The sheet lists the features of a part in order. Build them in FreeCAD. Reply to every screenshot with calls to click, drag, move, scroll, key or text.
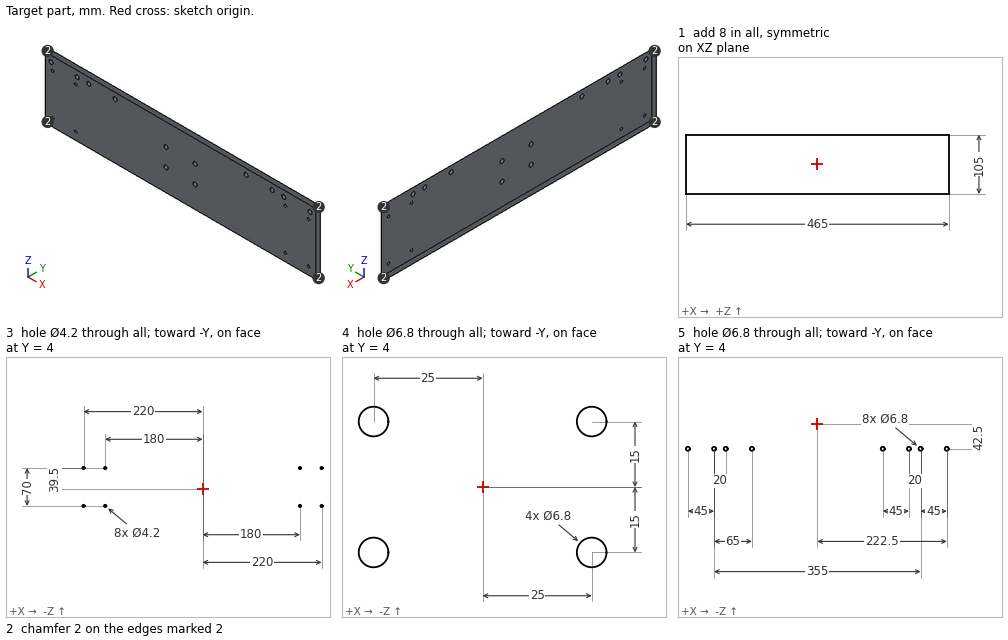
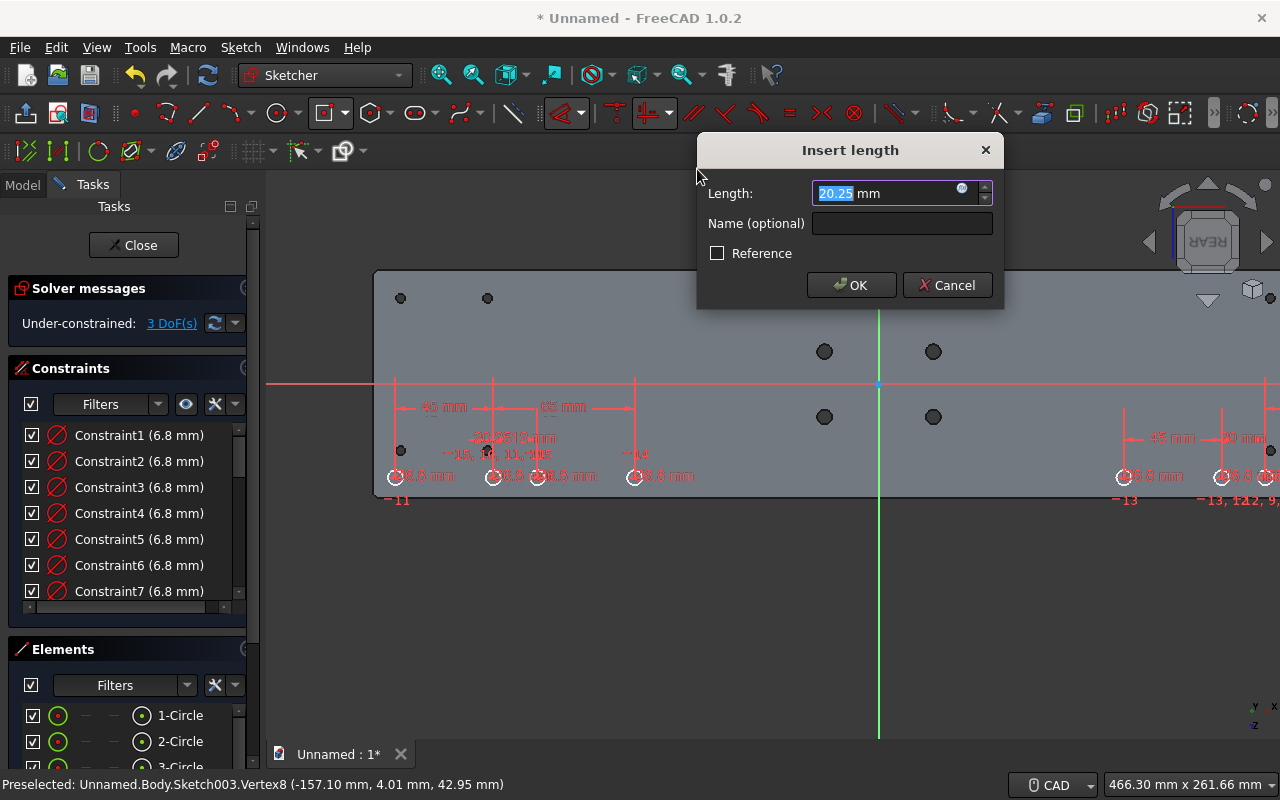
text(20)
key(Return)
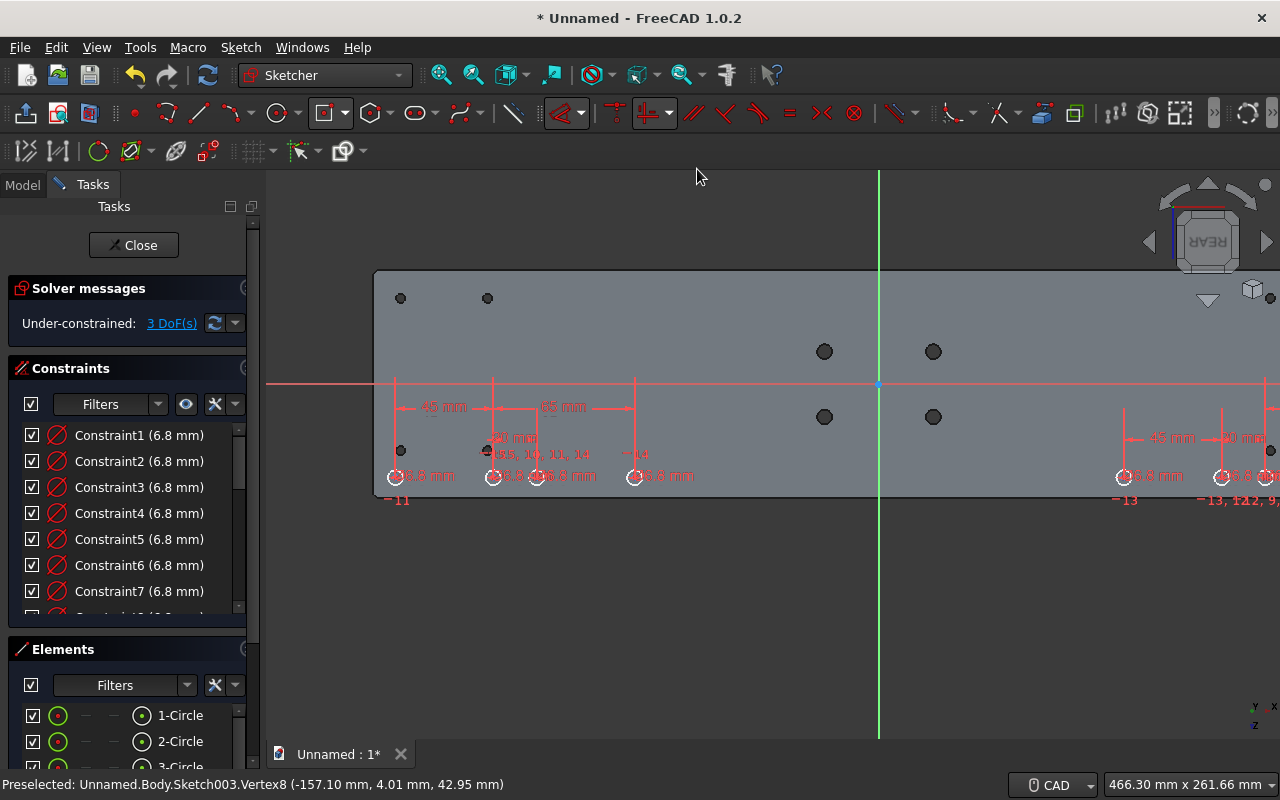
scroll(492, 479, down, 3)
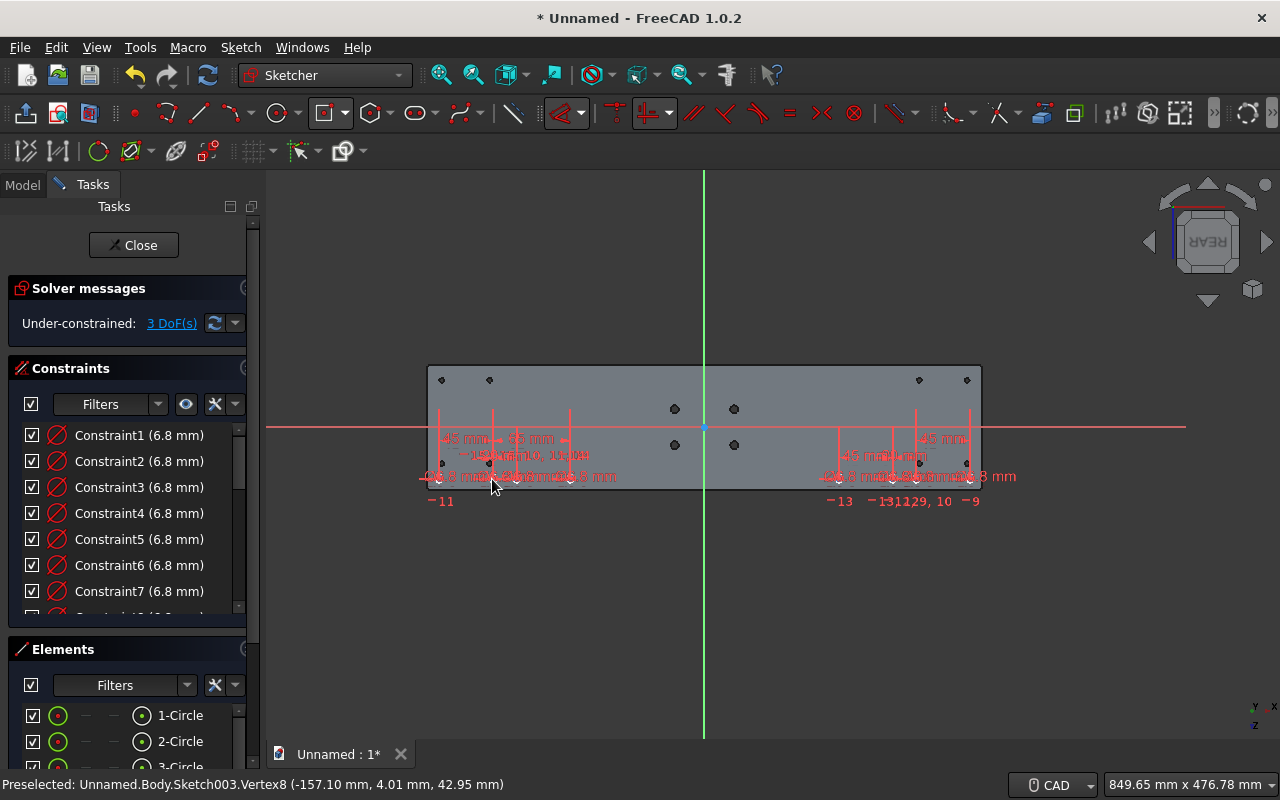
click(970, 479)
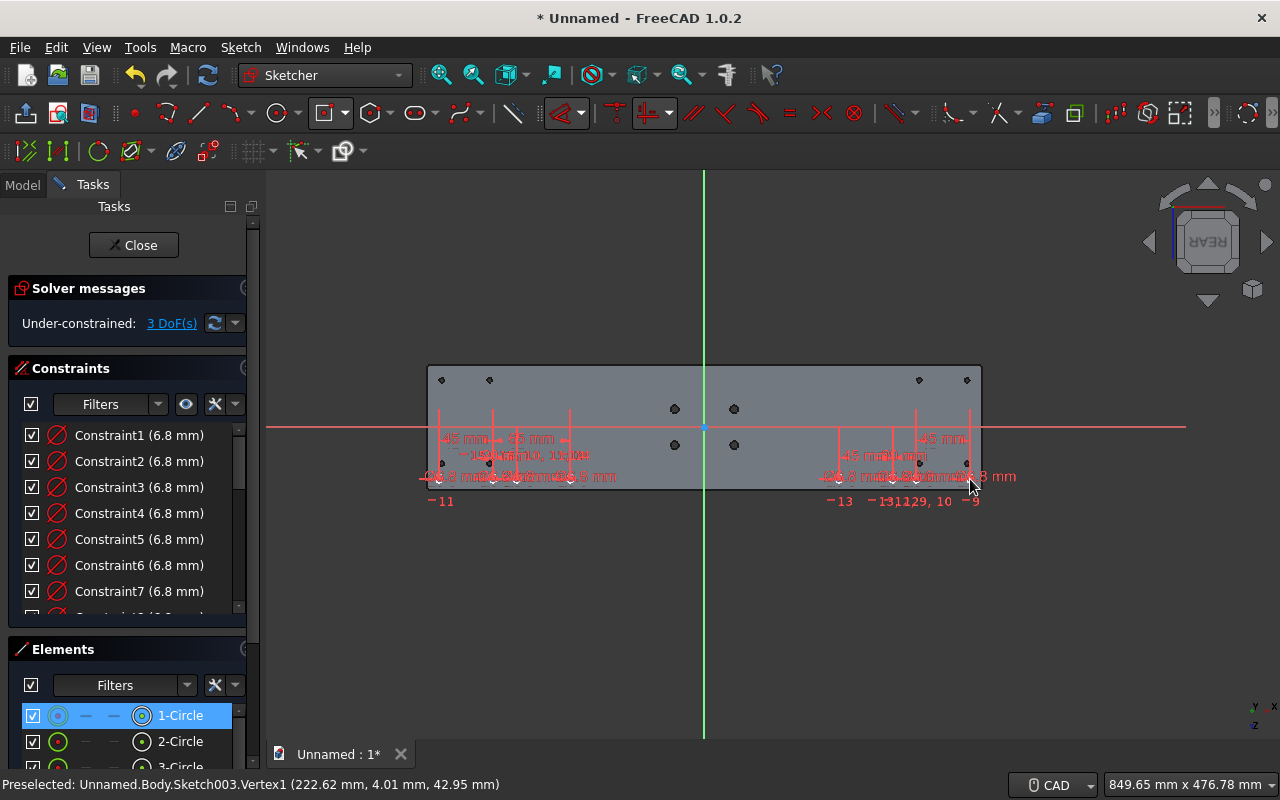
click(584, 114)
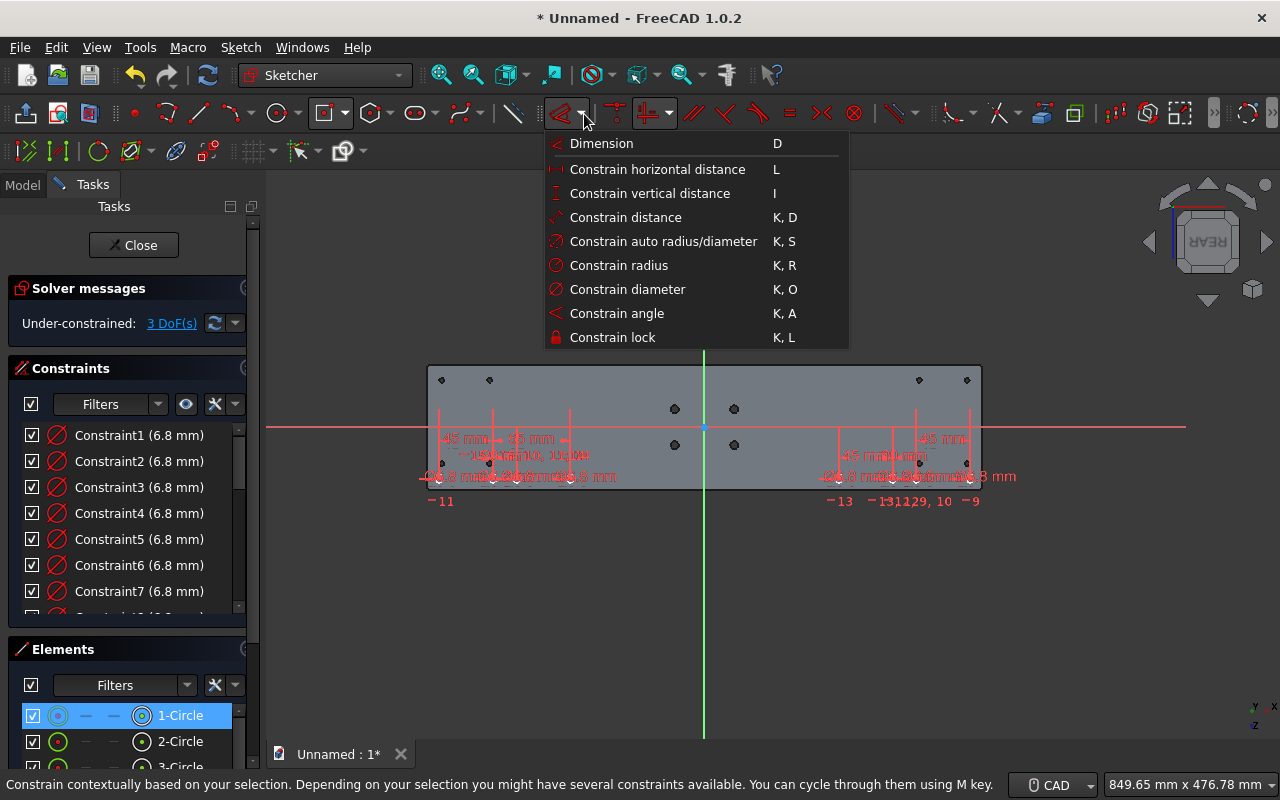
click(697, 193)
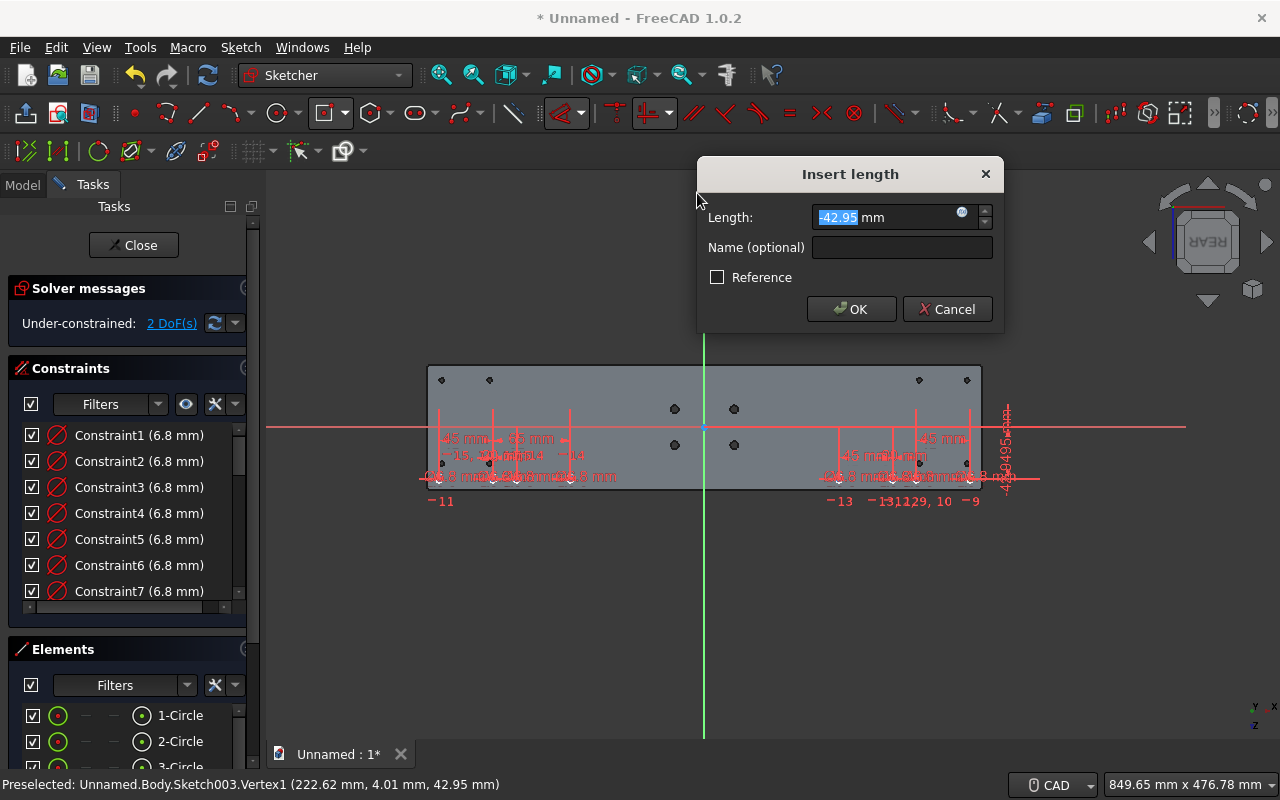
text(-42.5)
key(Return)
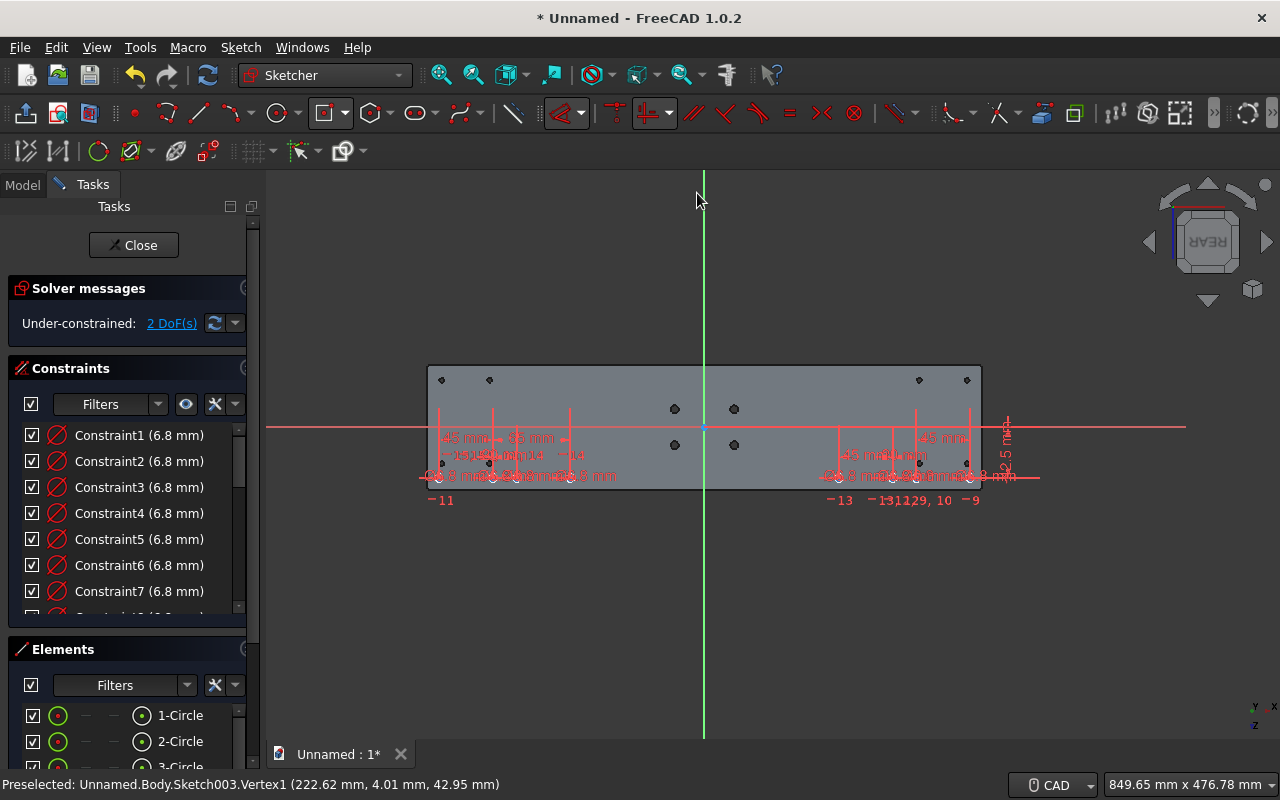
click(916, 478)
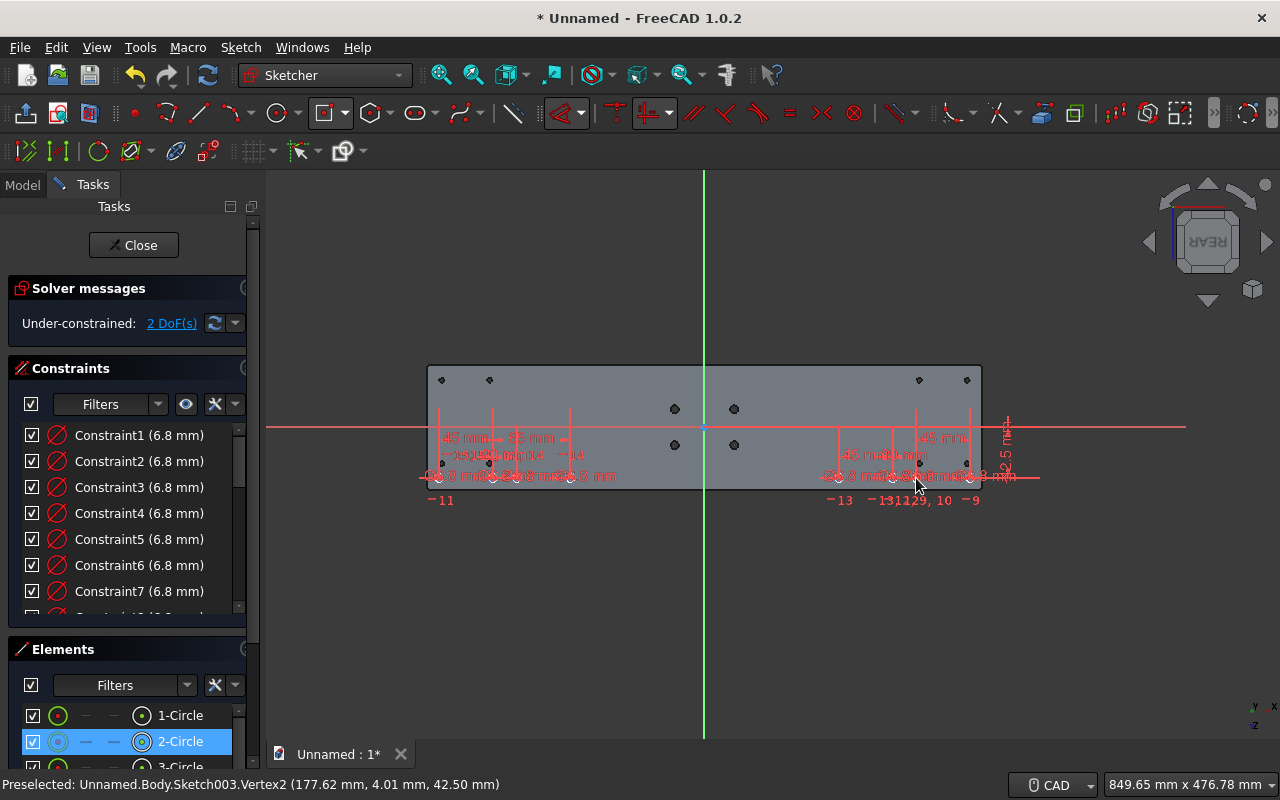
click(493, 478)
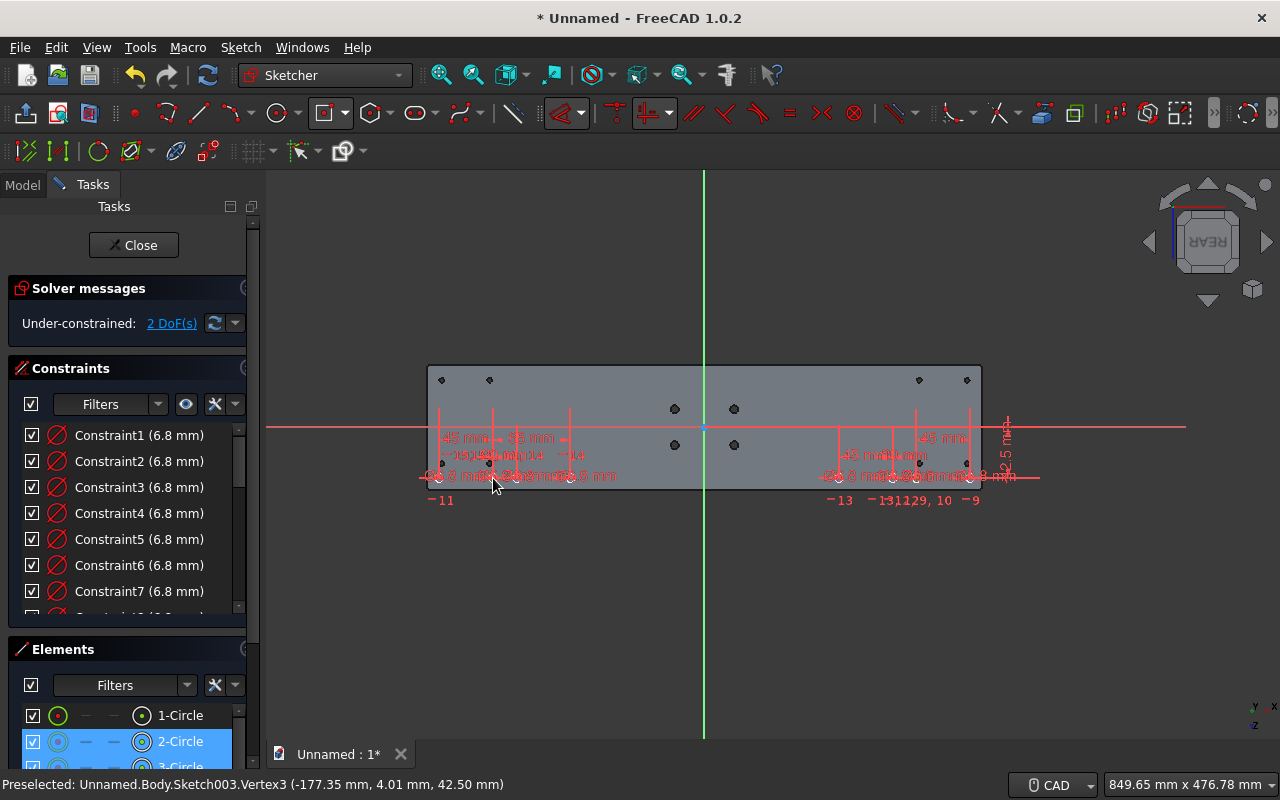
click(584, 114)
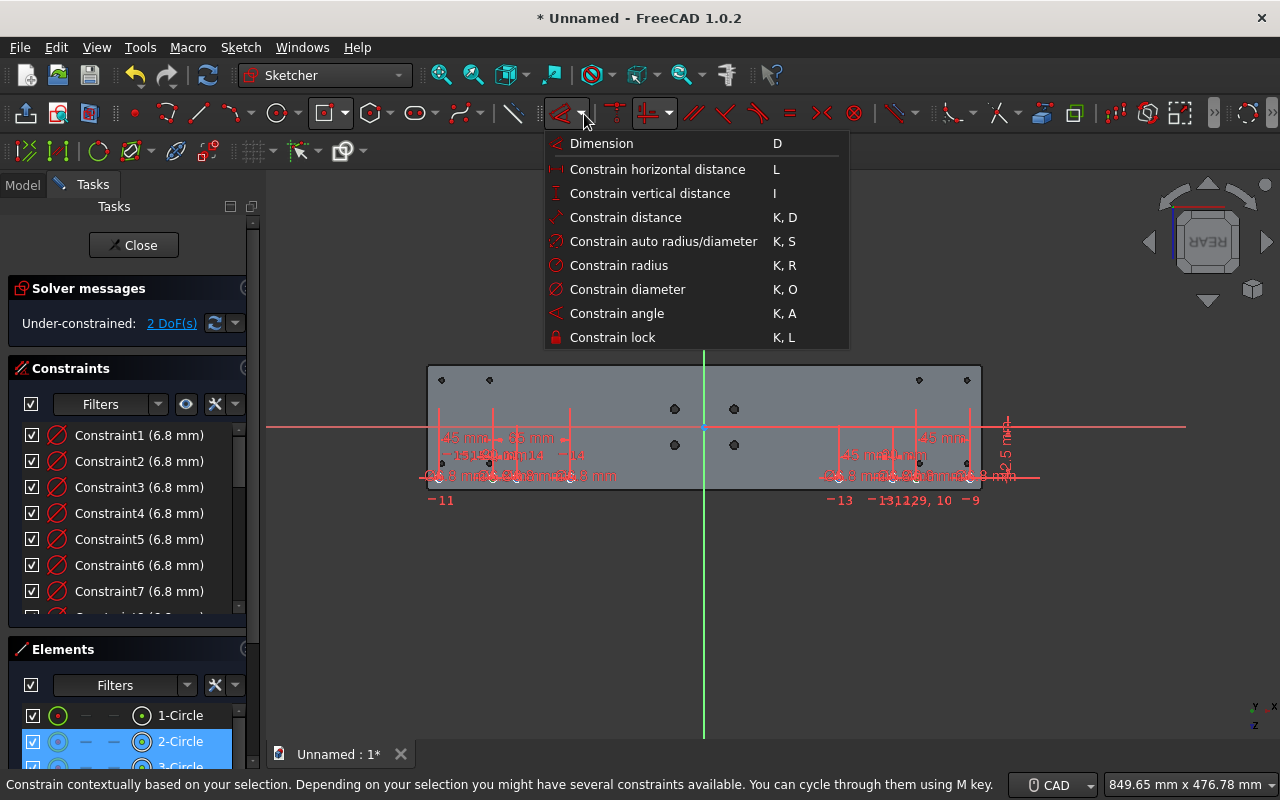
click(697, 169)